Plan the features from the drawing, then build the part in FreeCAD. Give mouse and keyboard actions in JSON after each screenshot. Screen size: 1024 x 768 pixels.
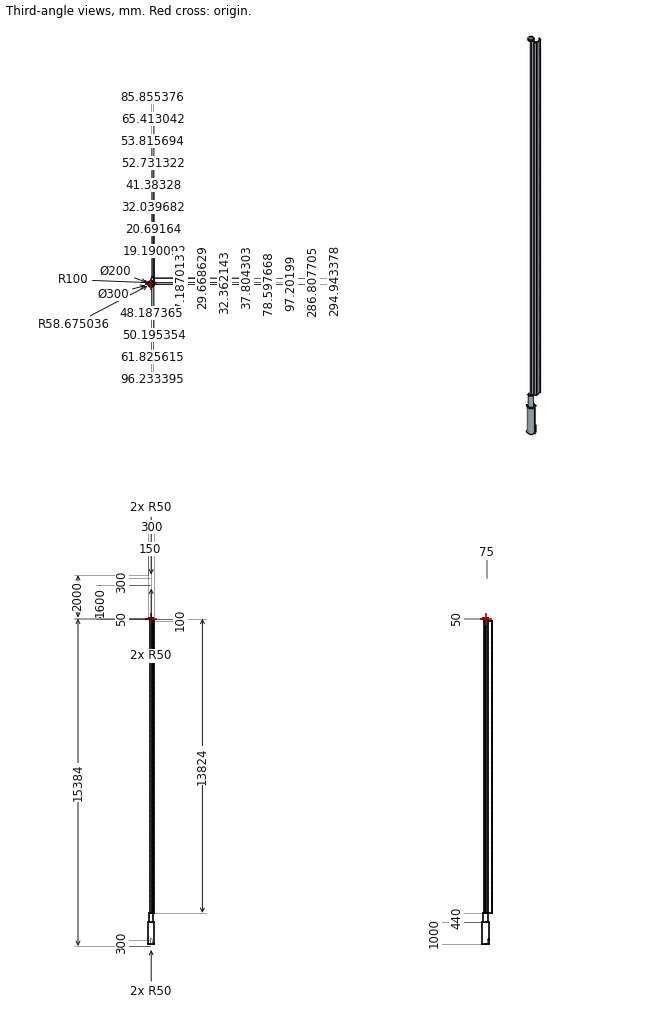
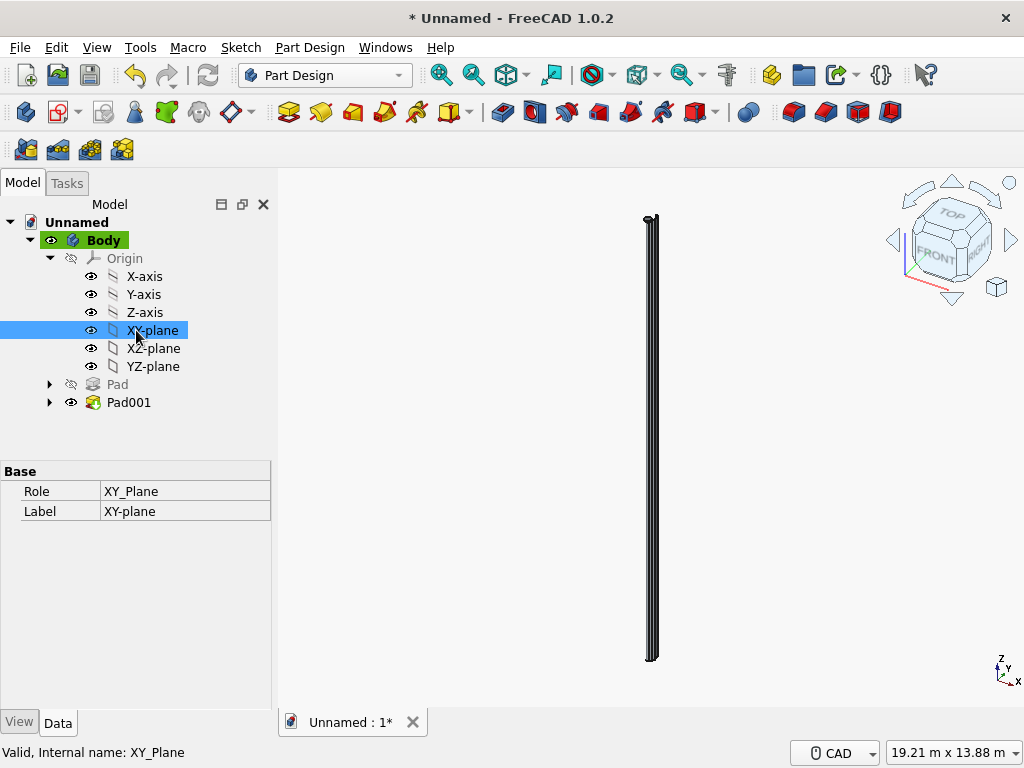
{"action": "left_click", "coordinate": [232, 112]}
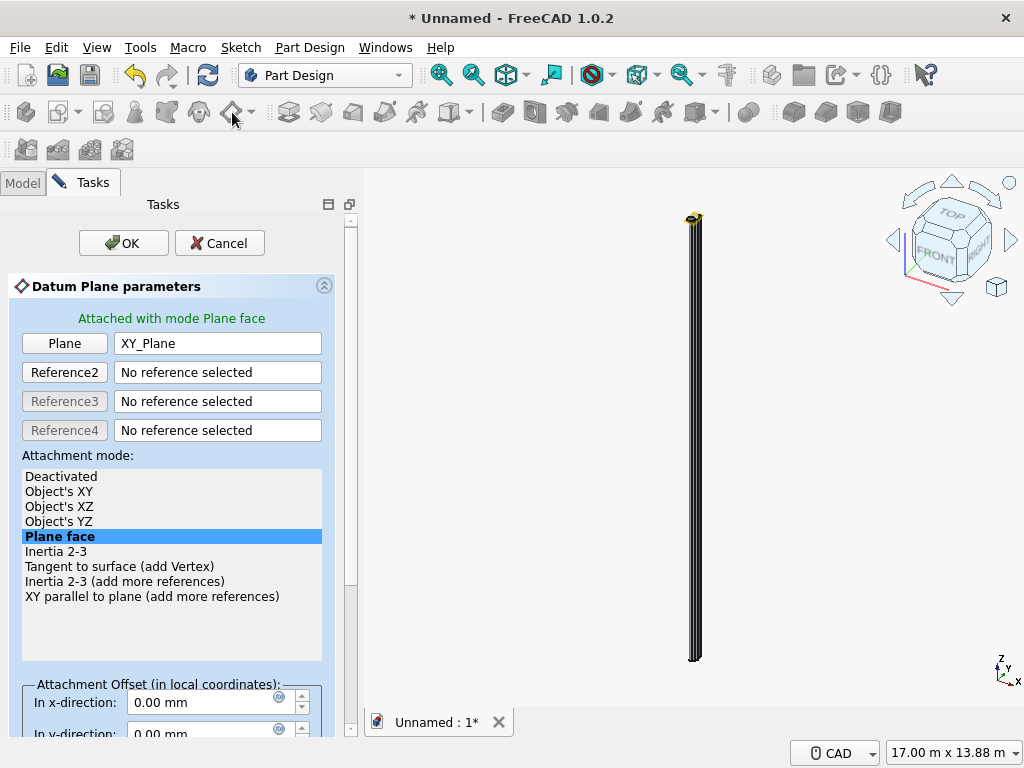
{"action": "scroll", "coordinate": [351, 475], "scroll_direction": "down", "scroll_amount": 2}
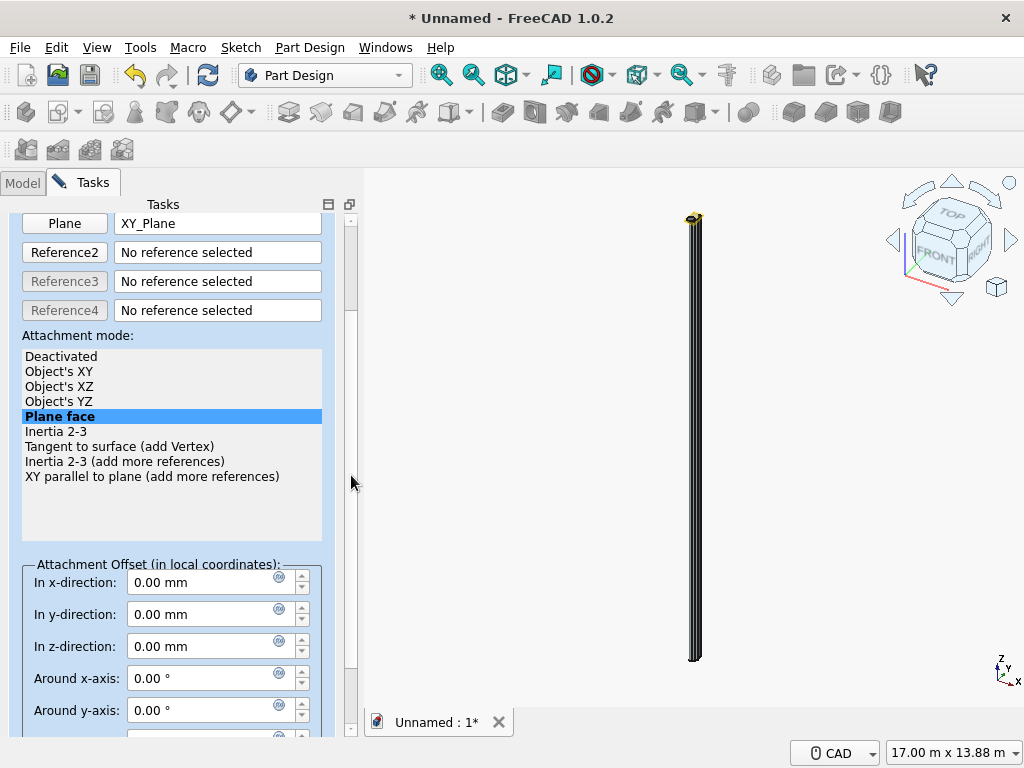
{"action": "triple_click", "coordinate": [210, 646]}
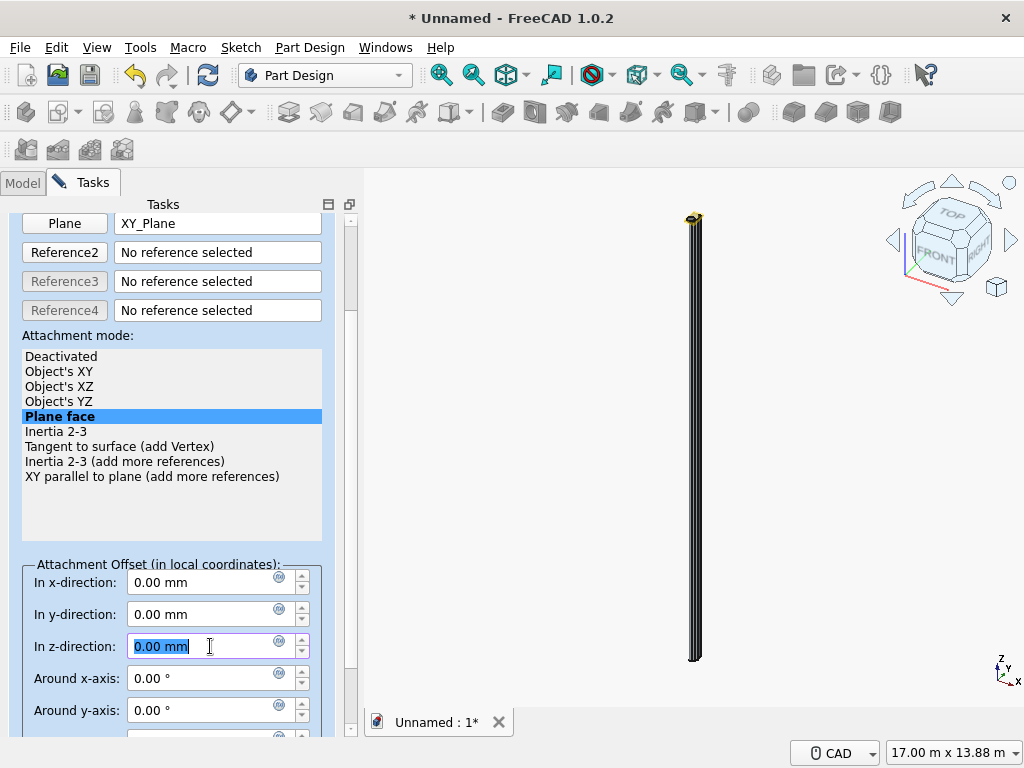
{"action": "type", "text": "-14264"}
{"action": "key", "text": "Tab"}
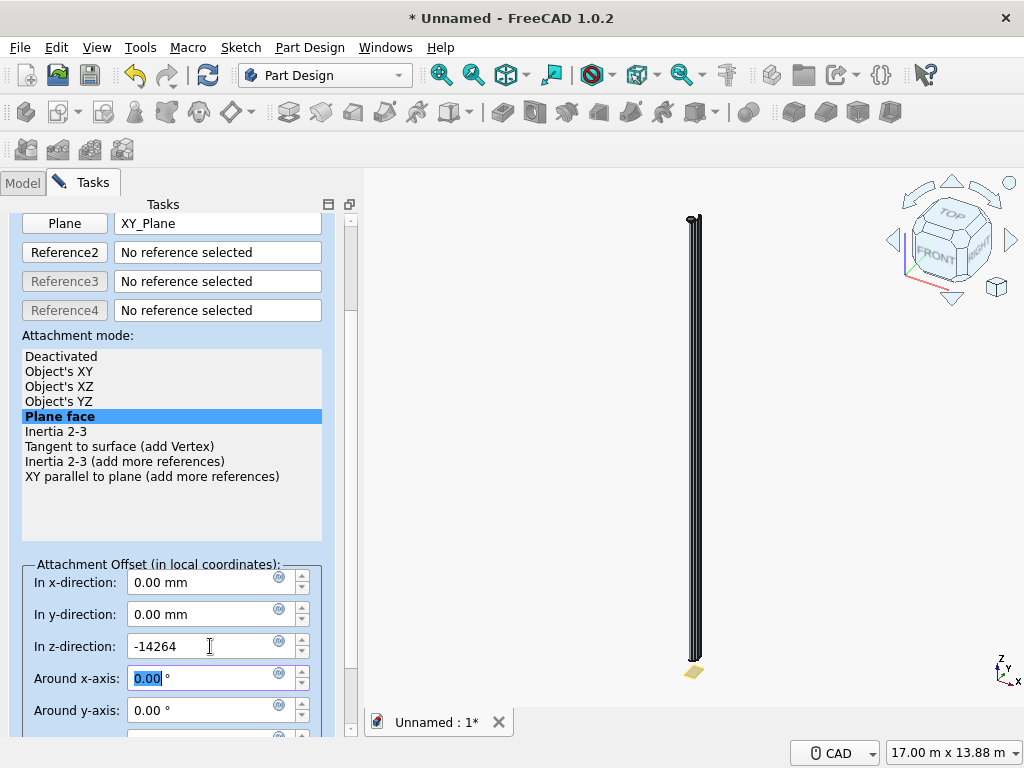
{"action": "scroll", "coordinate": [351, 475], "scroll_direction": "up", "scroll_amount": 3}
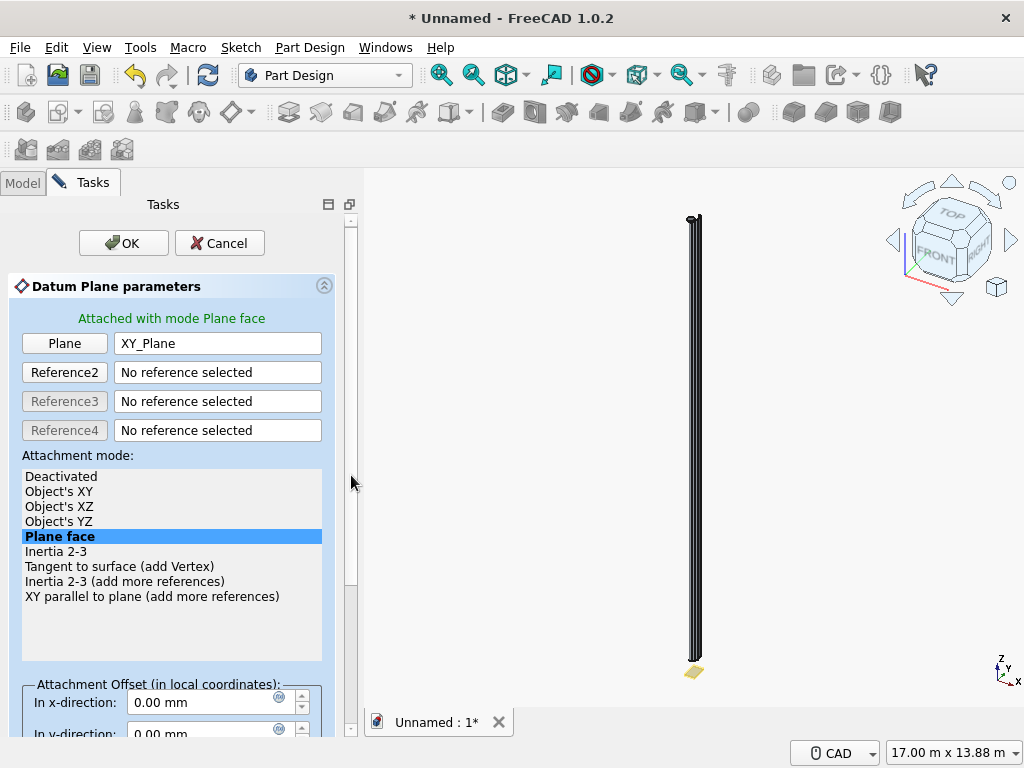
{"action": "left_click", "coordinate": [124, 243]}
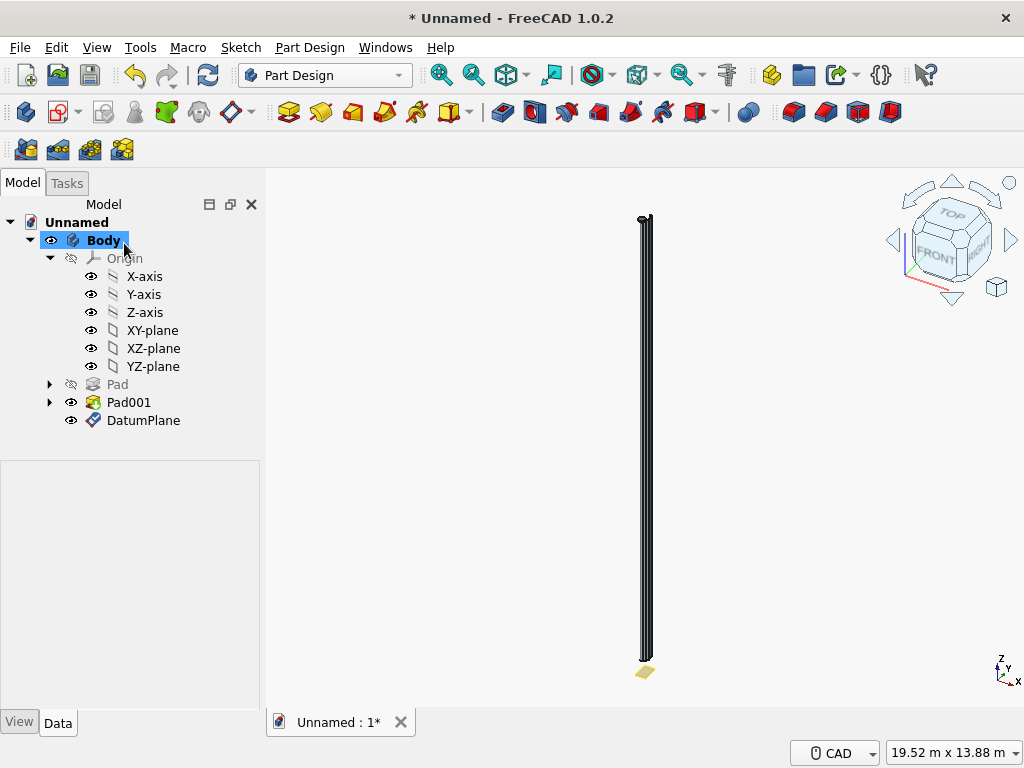
{"action": "left_click", "coordinate": [116, 420]}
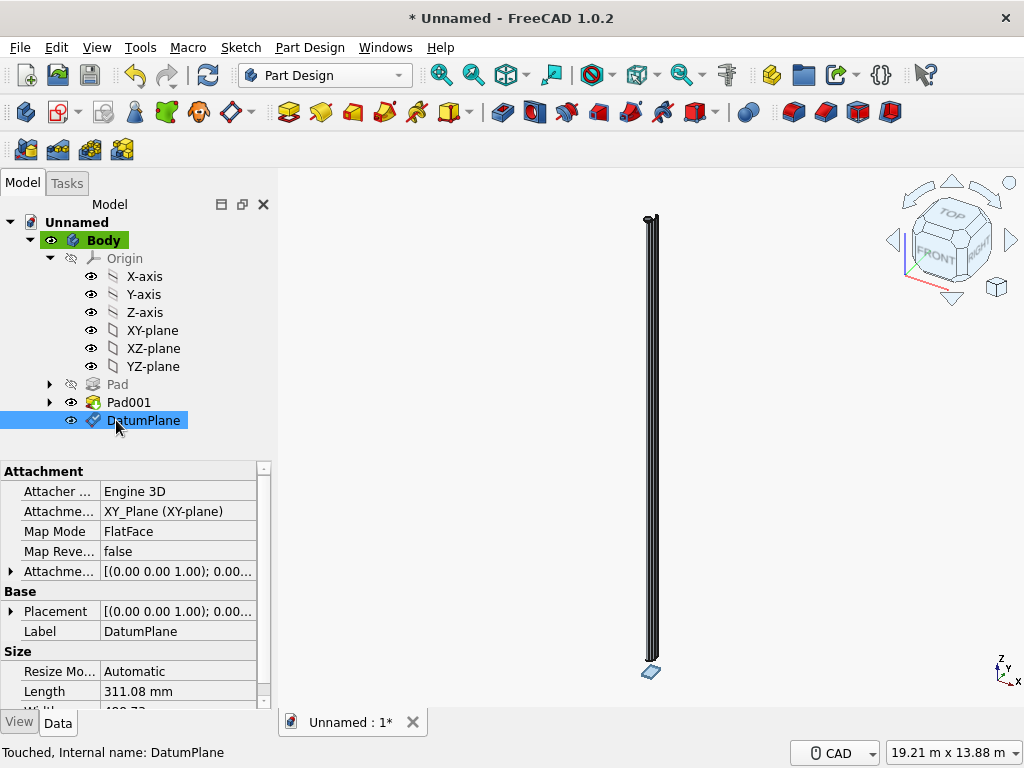
{"action": "left_click", "coordinate": [58, 112]}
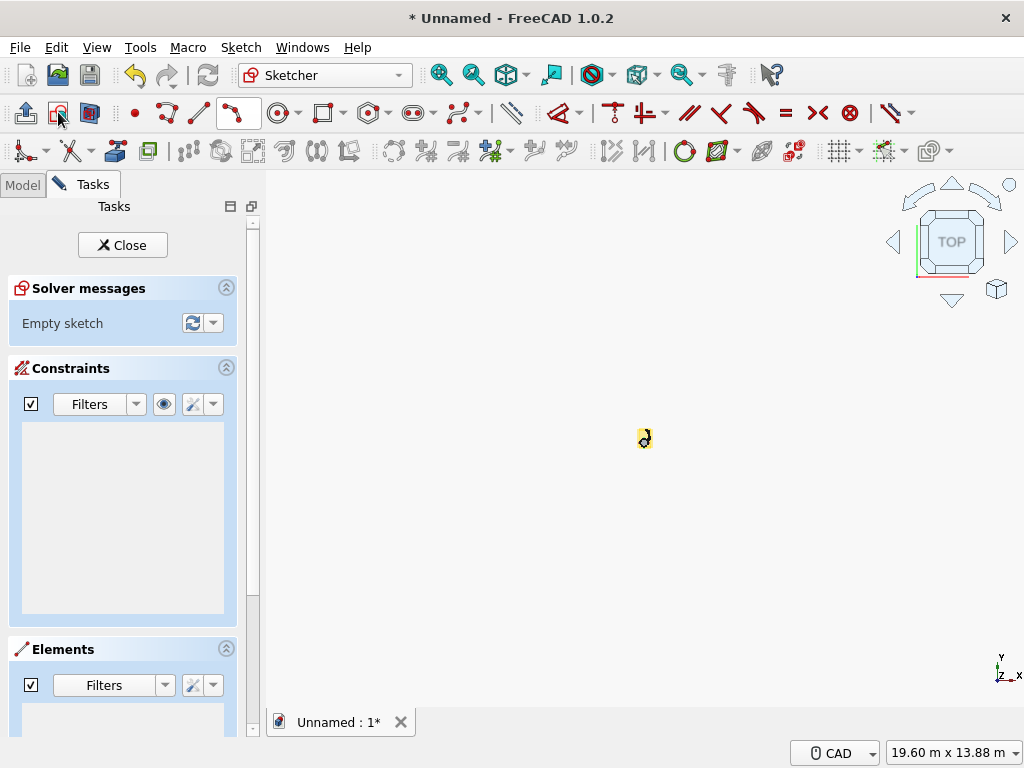
{"action": "left_click", "coordinate": [90, 114]}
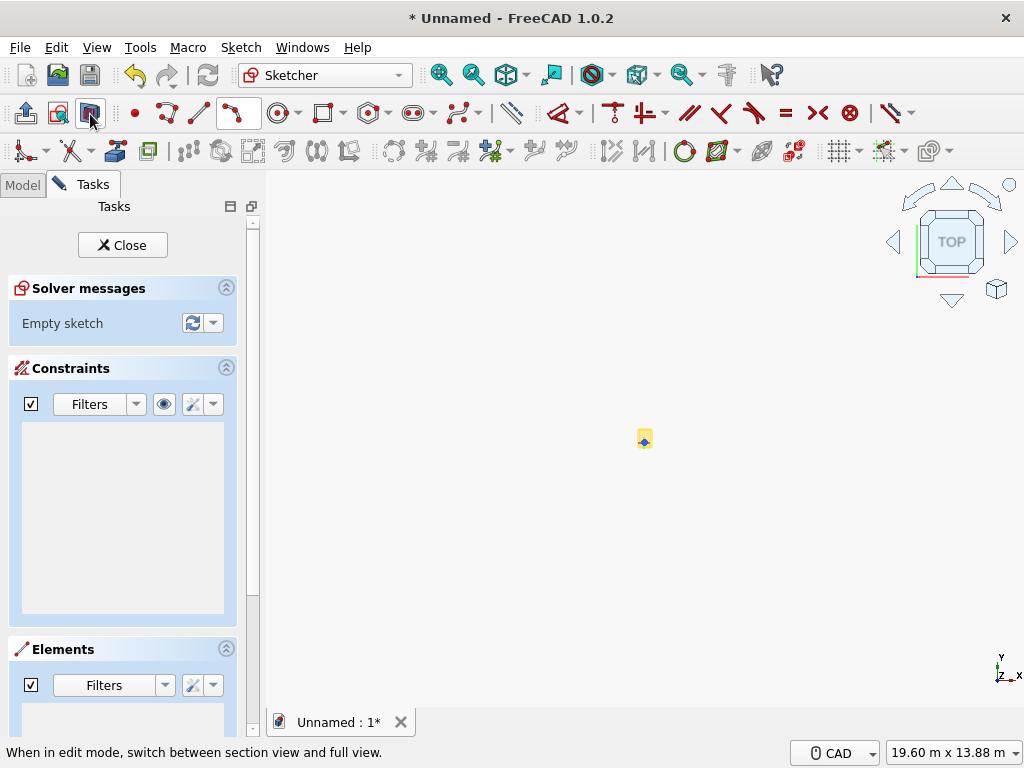
{"action": "scroll", "coordinate": [648, 443], "scroll_direction": "up", "scroll_amount": 15}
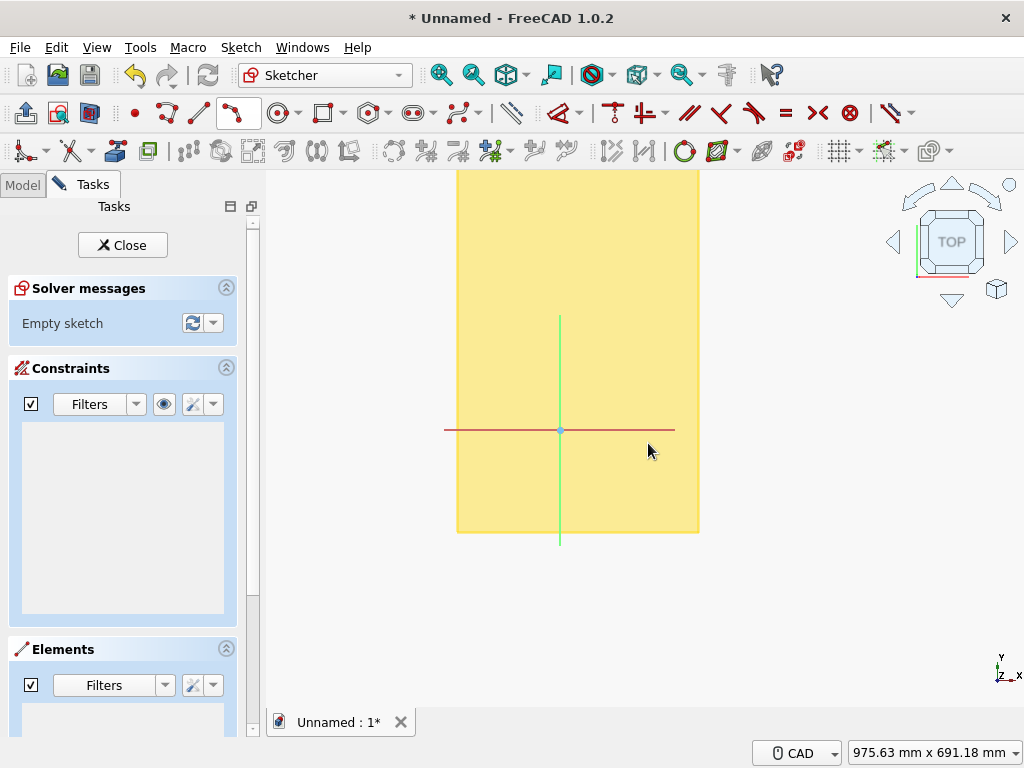
{"action": "scroll", "coordinate": [547, 424], "scroll_direction": "up", "scroll_amount": 4}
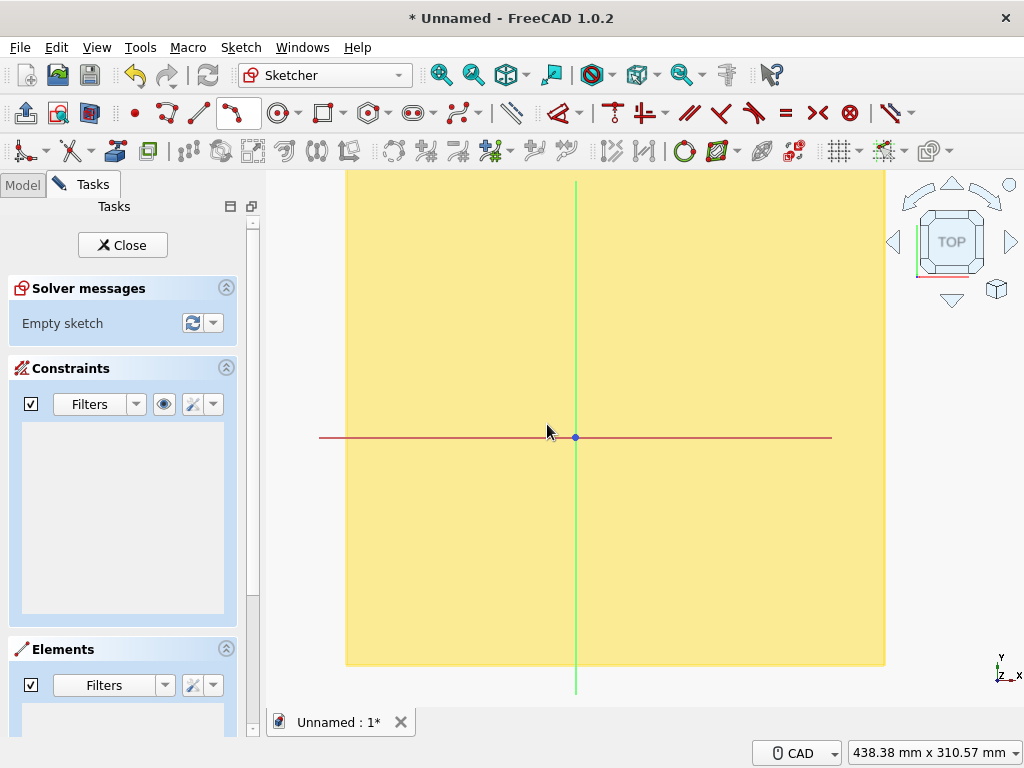
{"action": "left_click", "coordinate": [278, 114]}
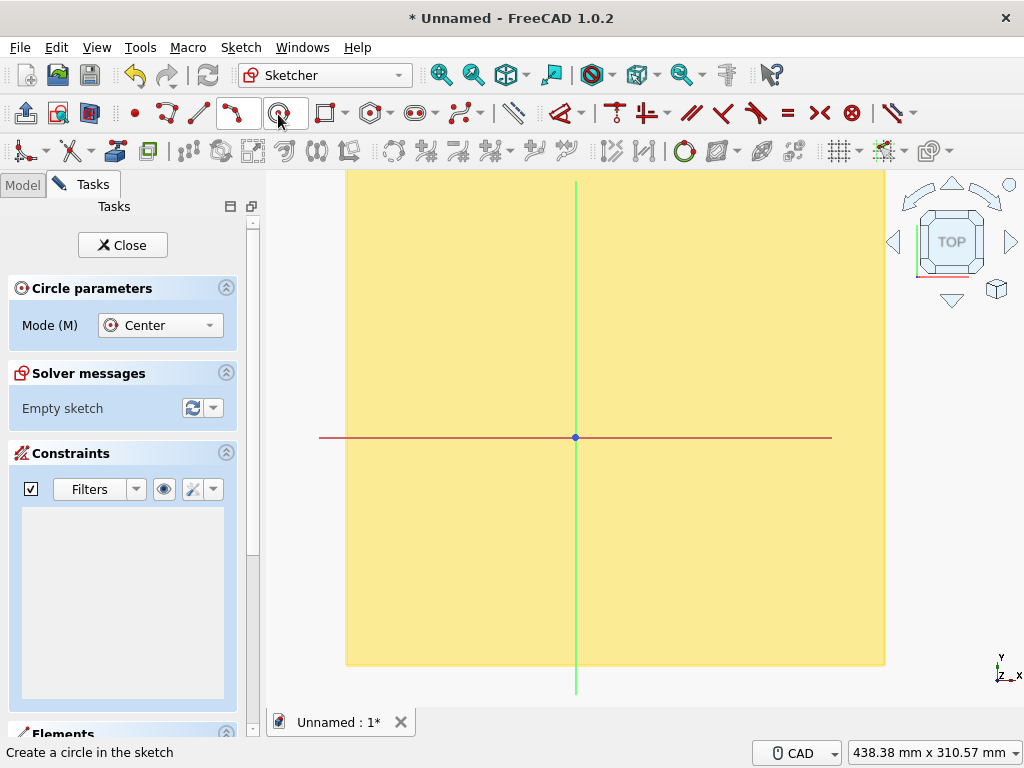
{"action": "left_click", "coordinate": [576, 438]}
{"action": "left_click", "coordinate": [698, 315]}
{"action": "key", "text": "Escape"}